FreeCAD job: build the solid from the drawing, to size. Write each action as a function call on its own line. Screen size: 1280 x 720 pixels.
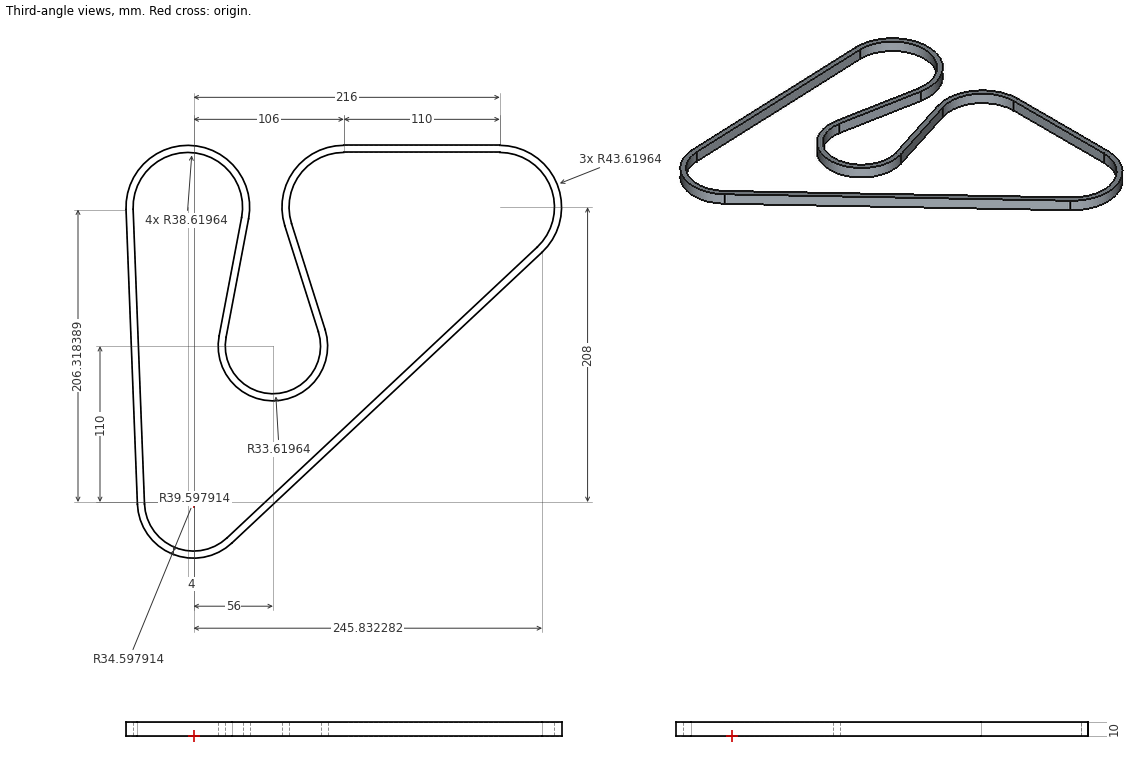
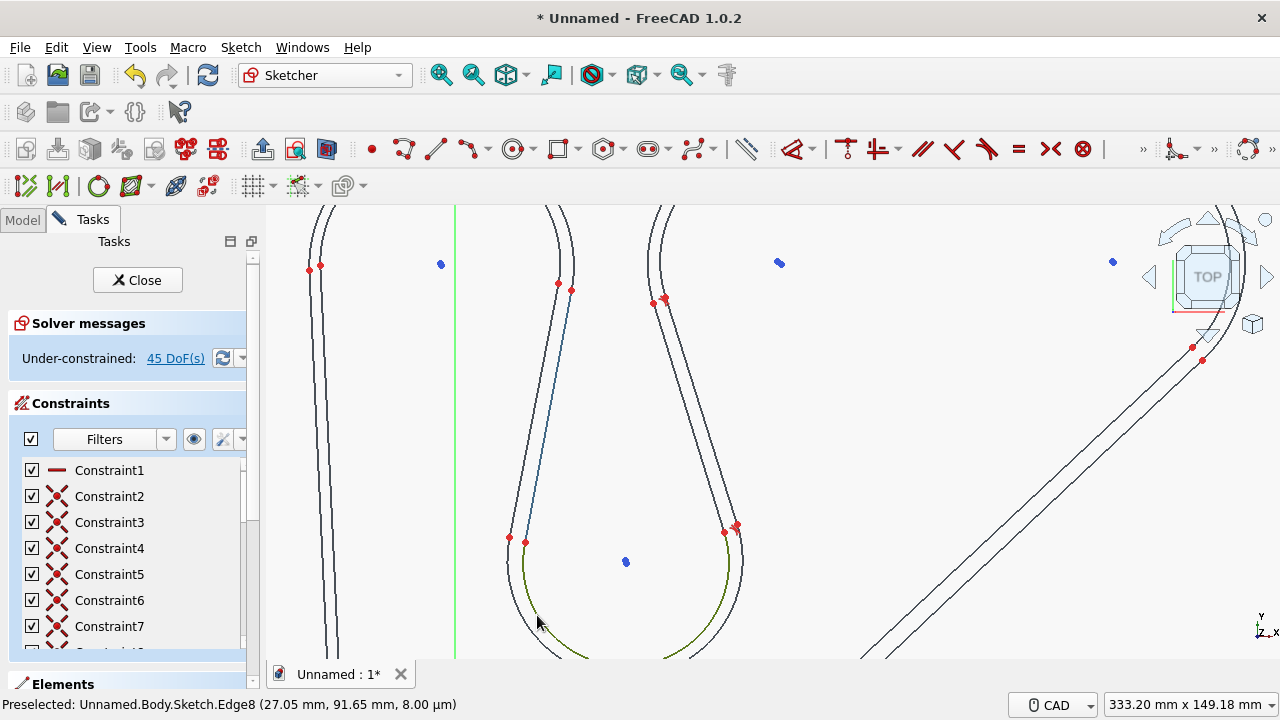
click(988, 150)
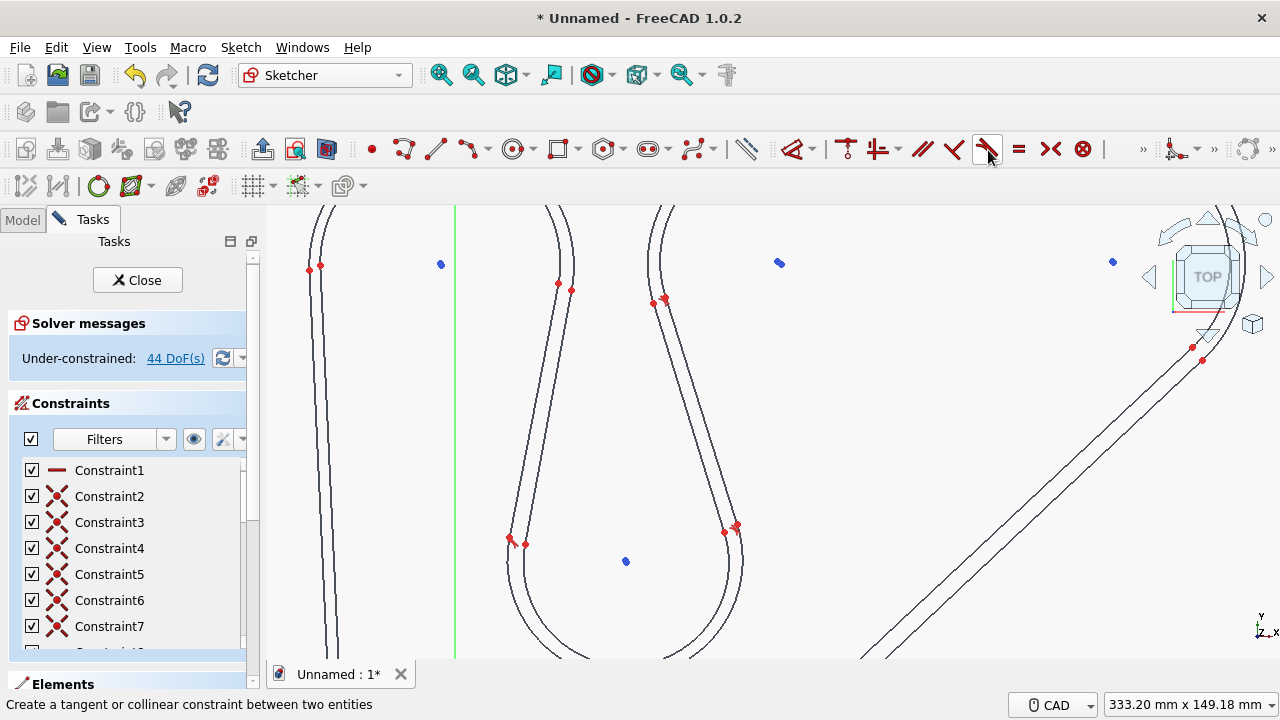
click(539, 468)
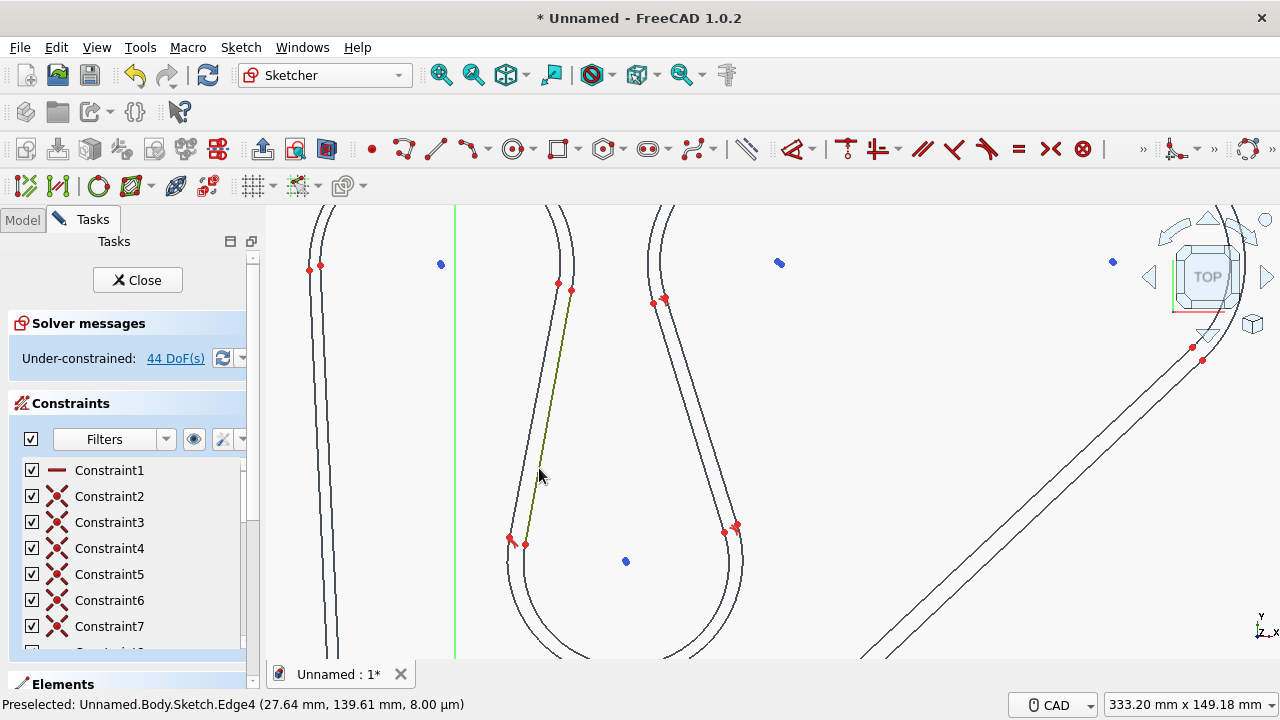
scroll(675, 374, down, 6)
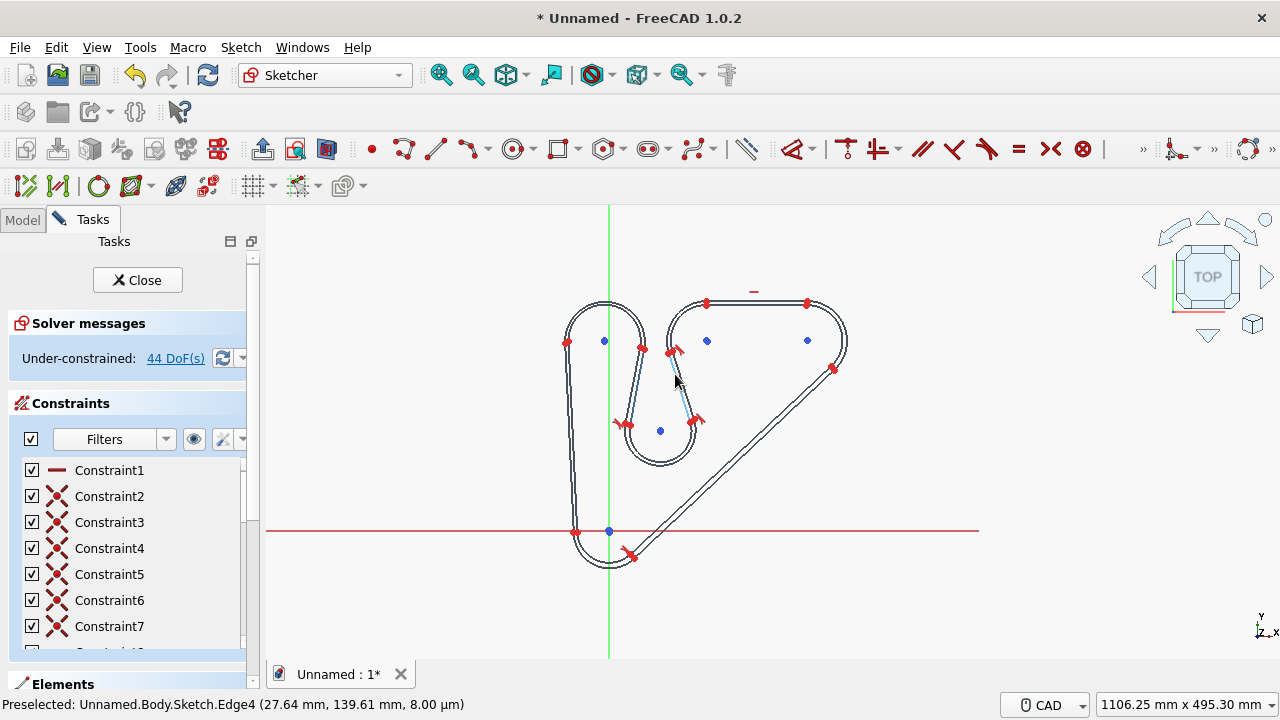
scroll(632, 312, up, 8)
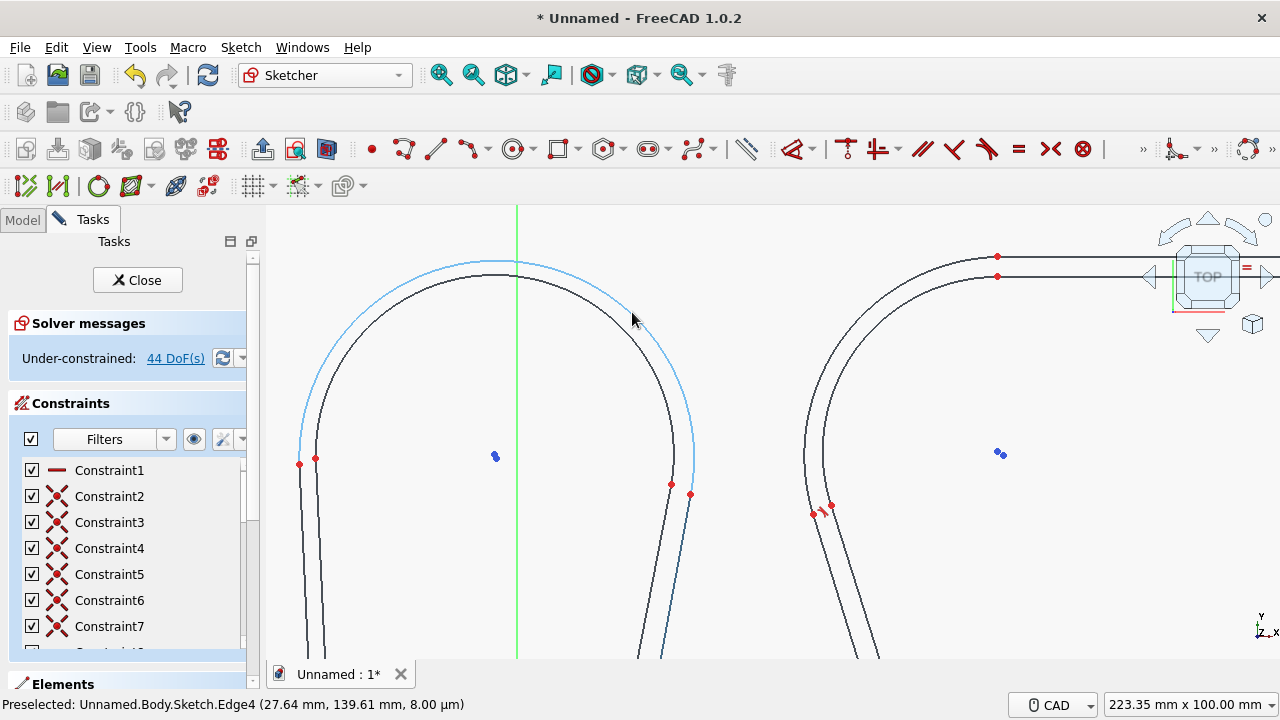
click(631, 313)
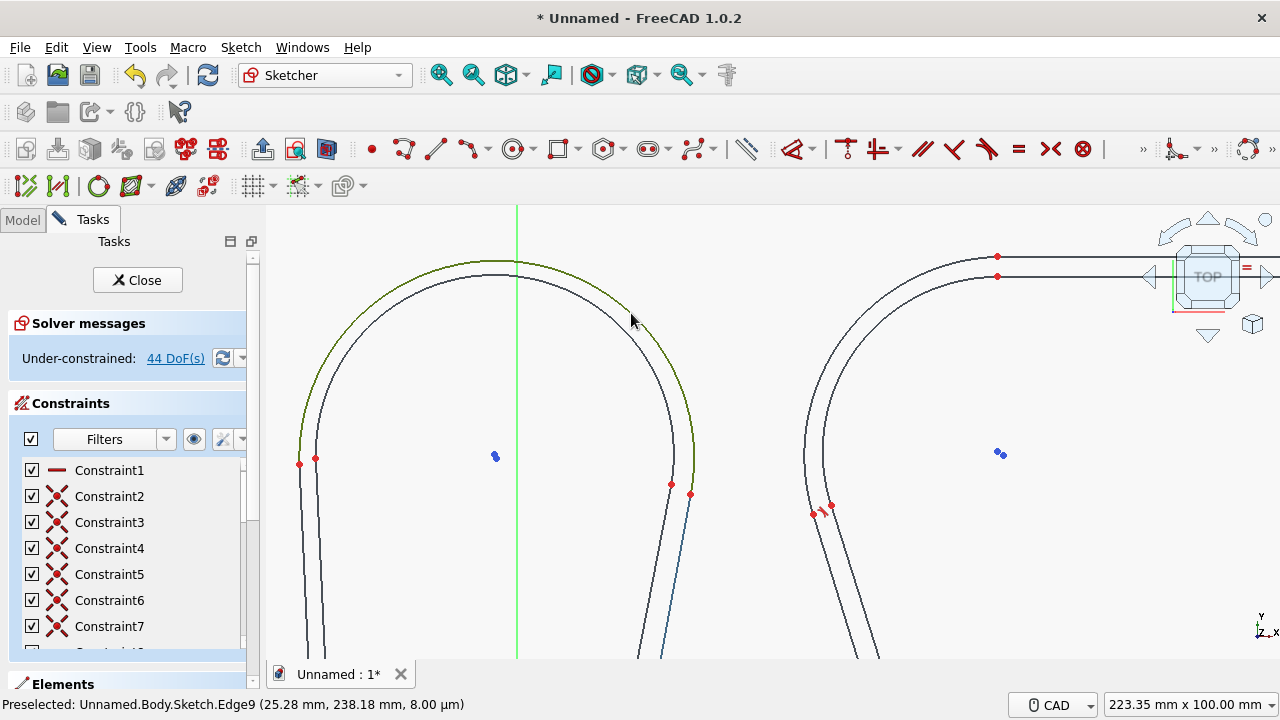
click(988, 150)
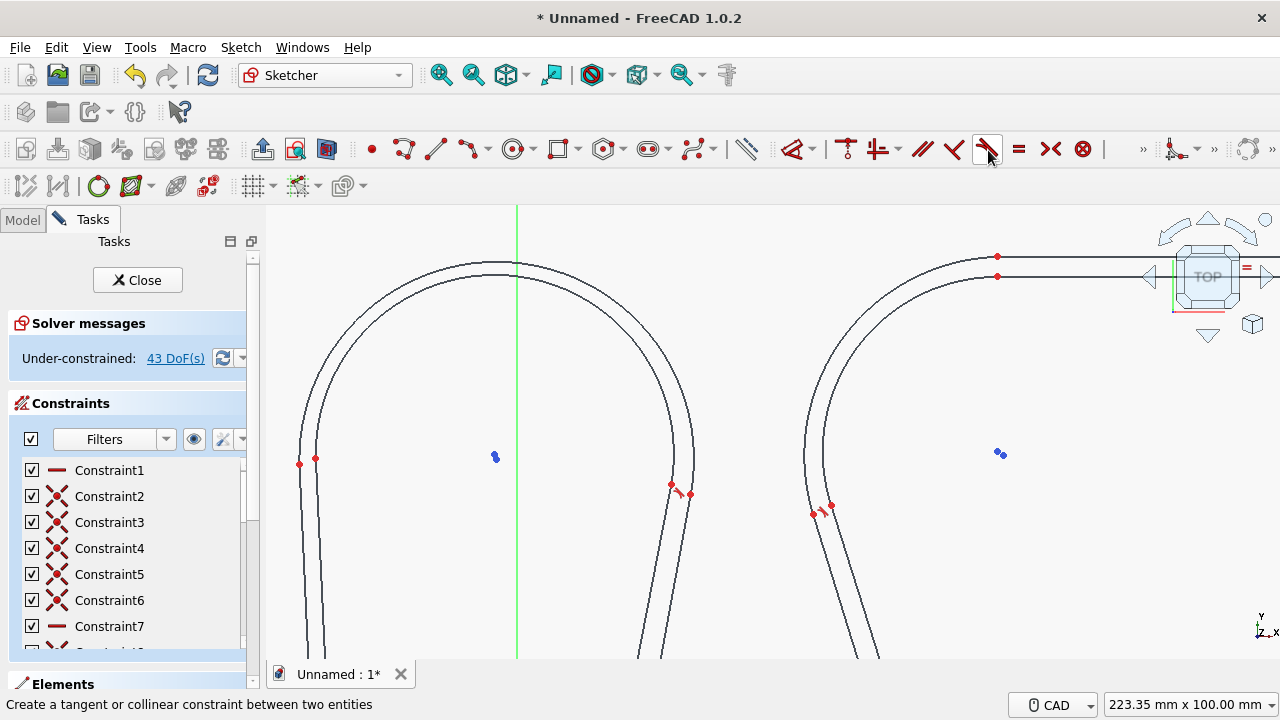
scroll(632, 312, down, 8)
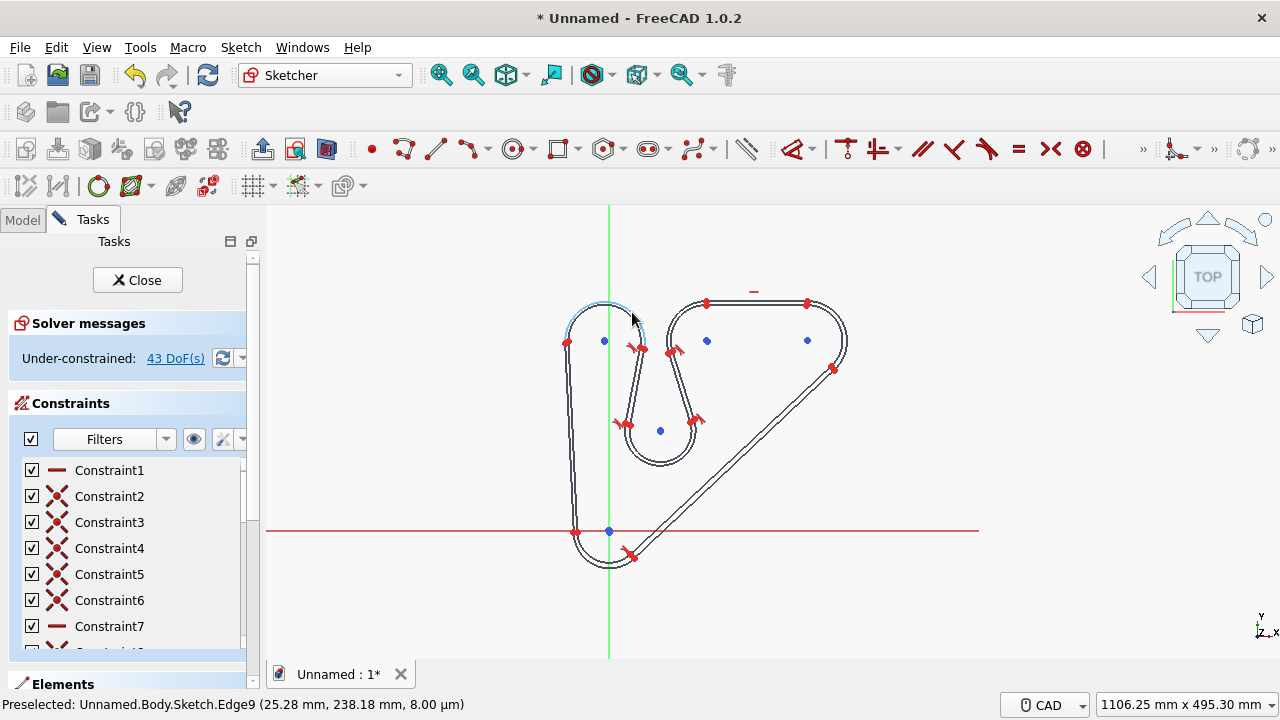
scroll(568, 400, up, 8)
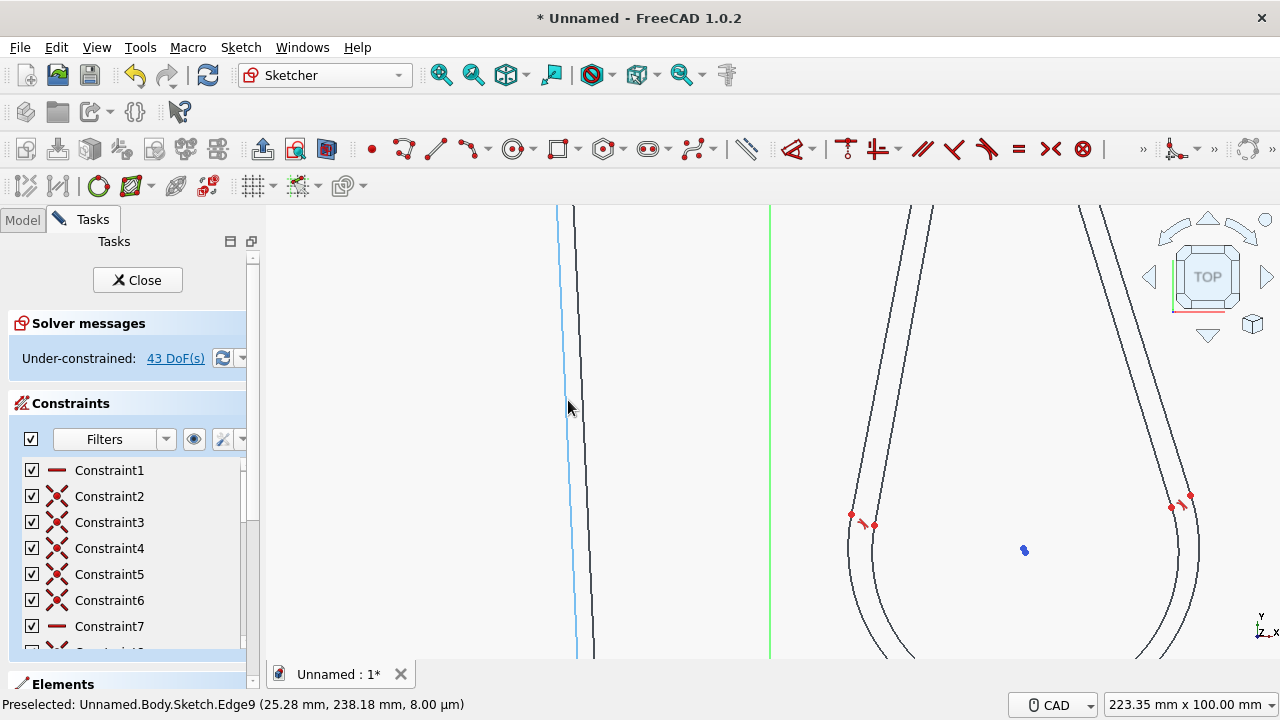
click(566, 397)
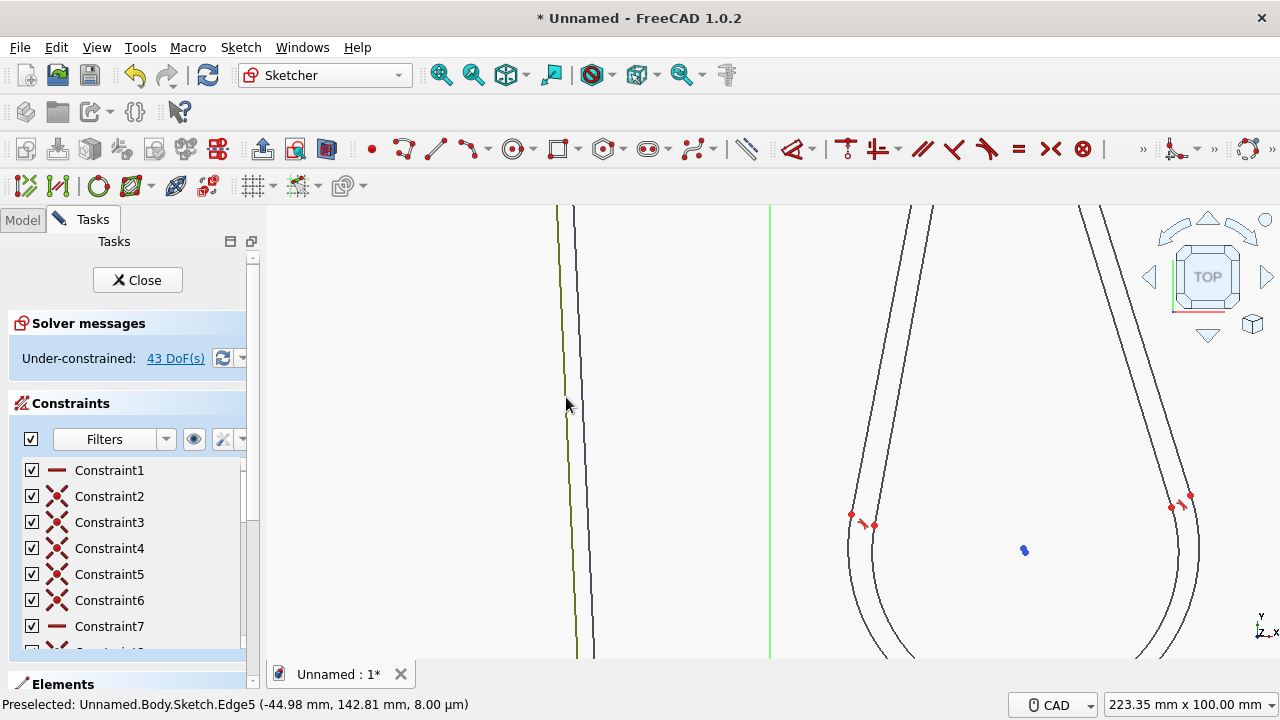
scroll(568, 400, down, 8)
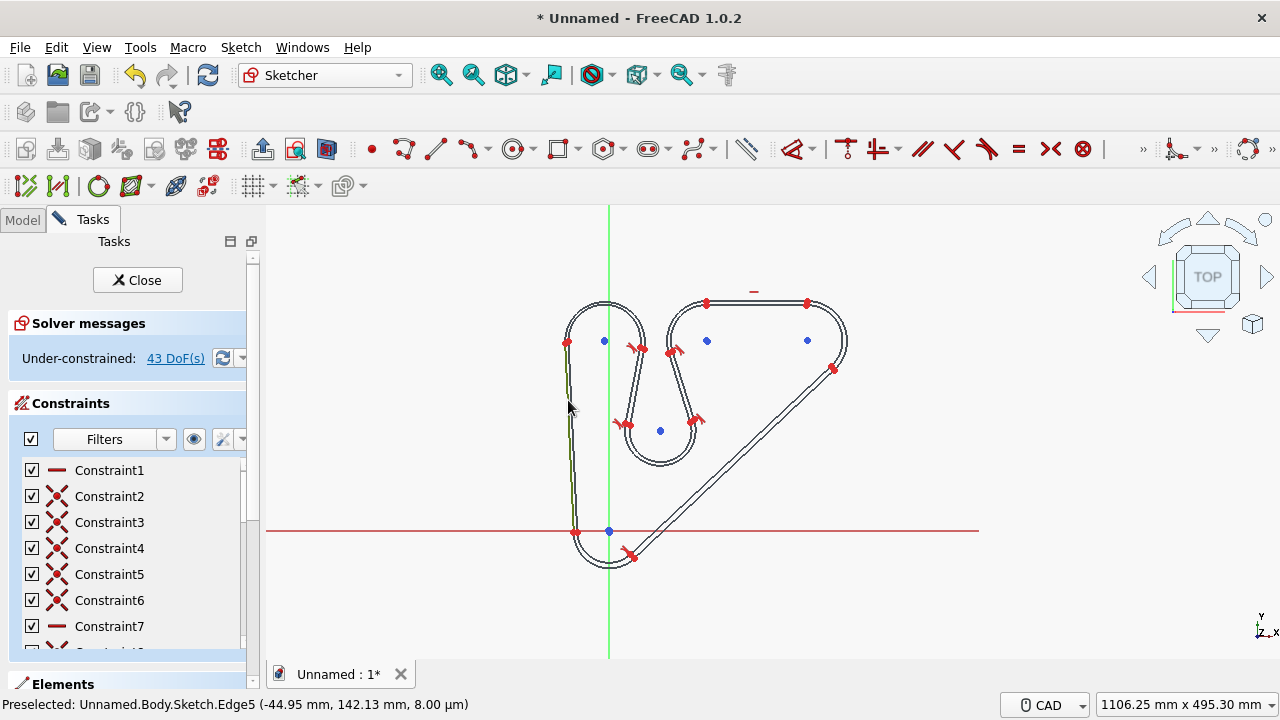
scroll(582, 555, up, 6)